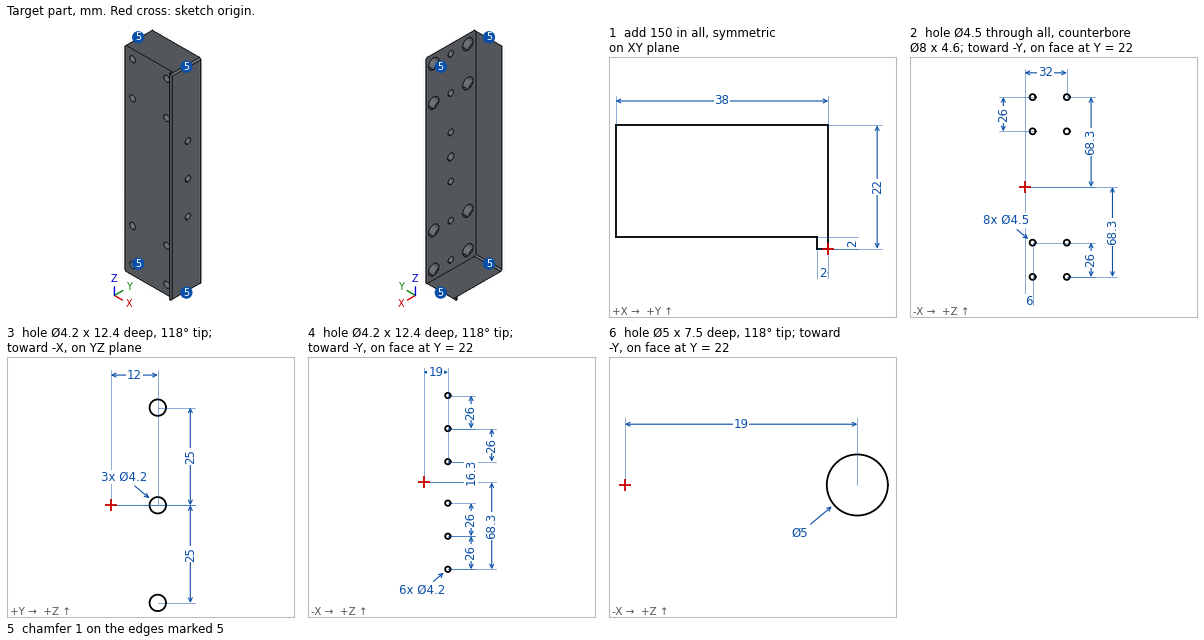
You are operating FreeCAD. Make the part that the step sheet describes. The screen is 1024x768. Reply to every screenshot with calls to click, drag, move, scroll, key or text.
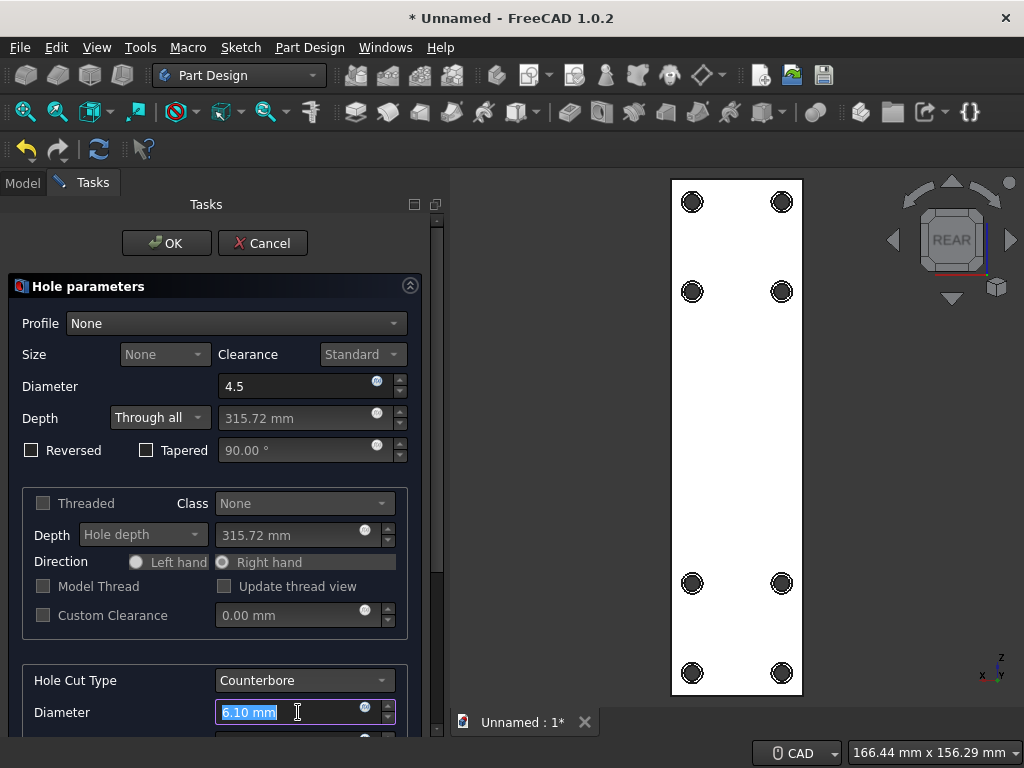
text(8)
key(Tab)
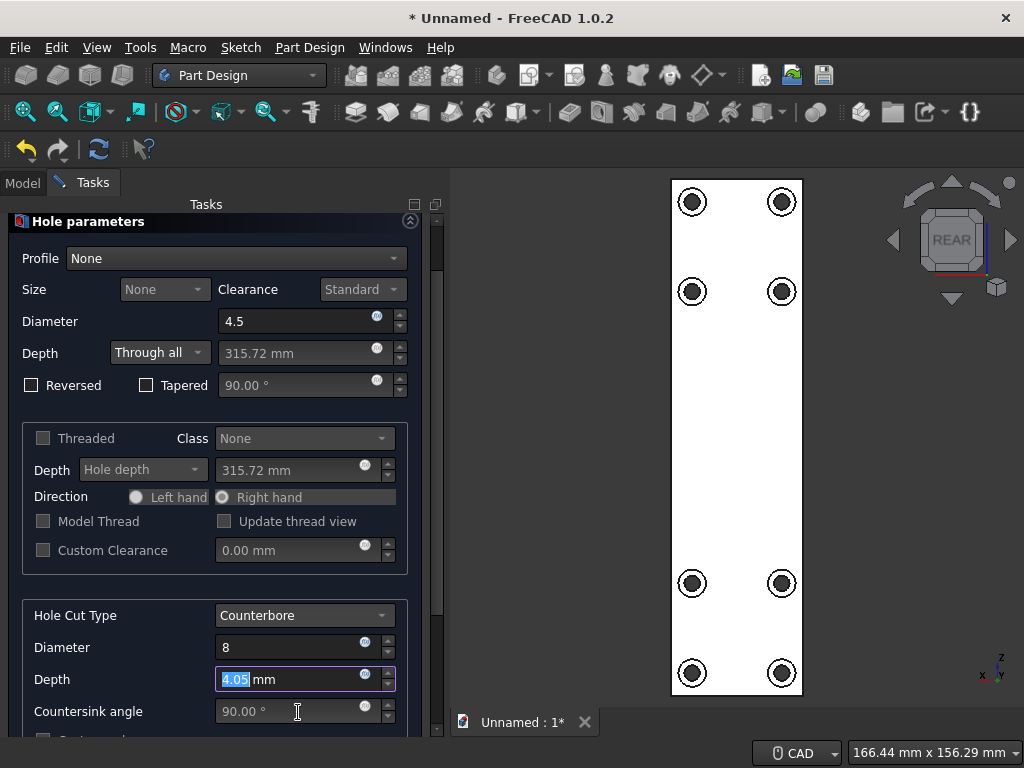
text(4.6)
key(Tab)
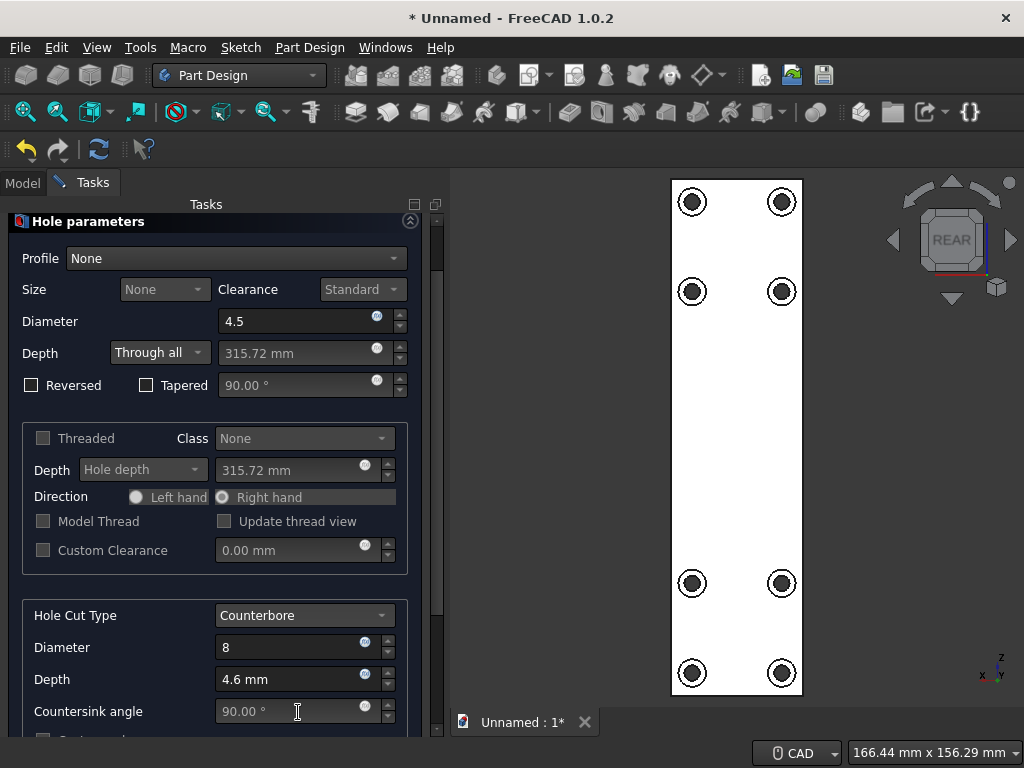
scroll(437, 475, up, 2)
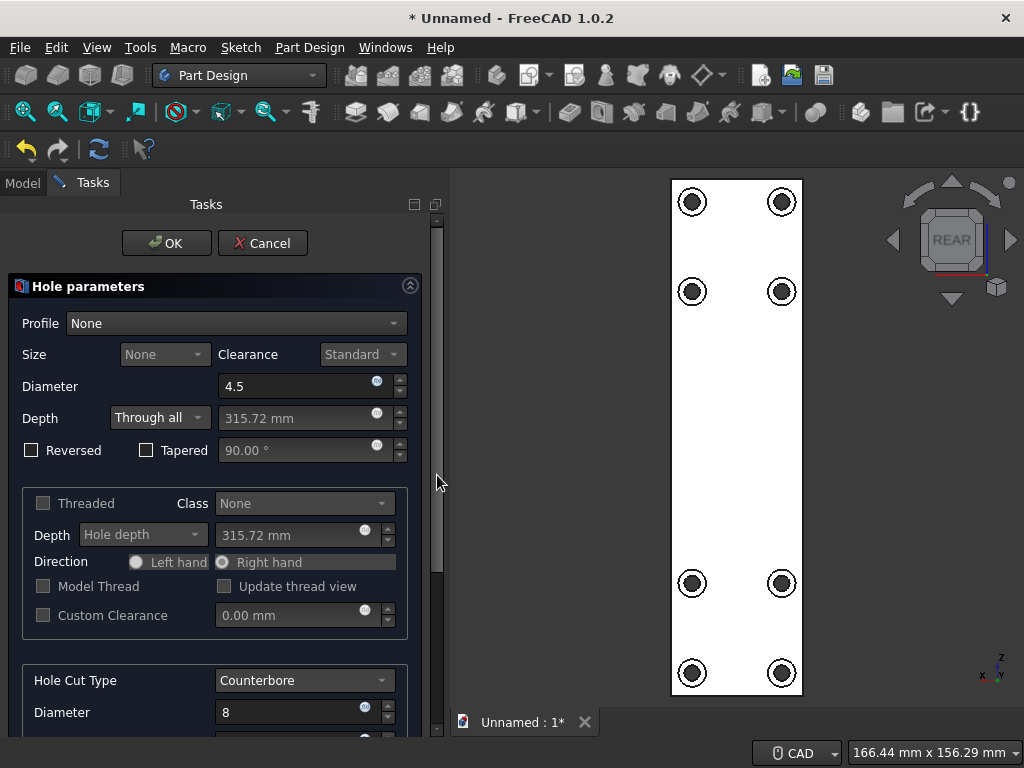
click(167, 243)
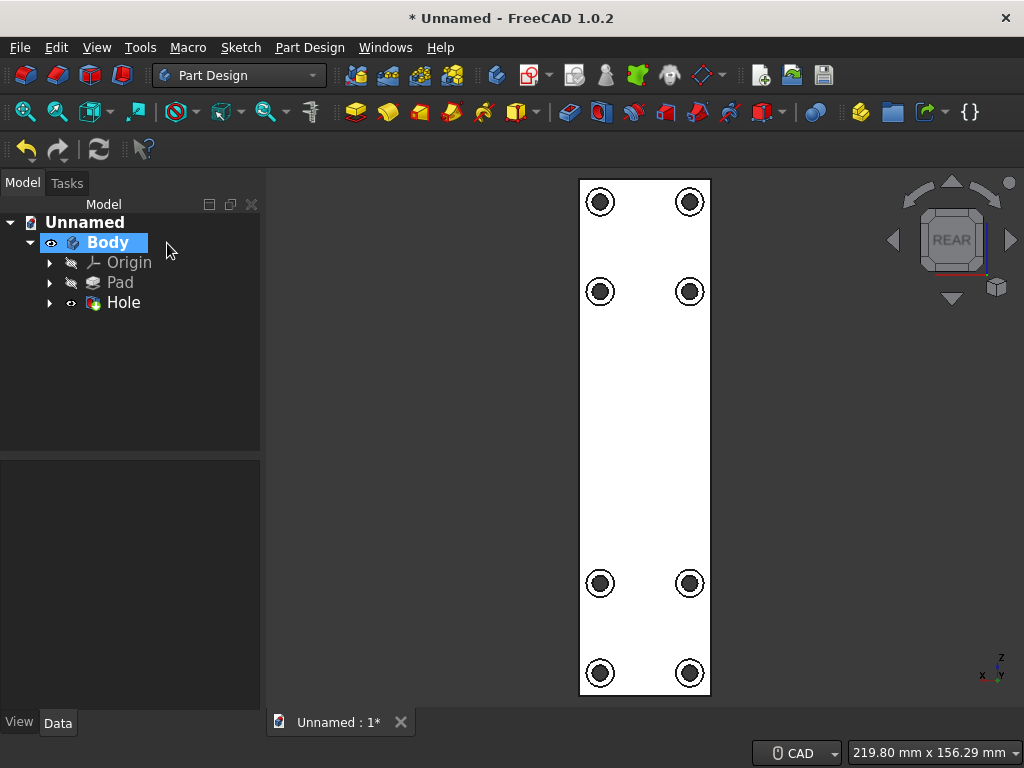
click(530, 76)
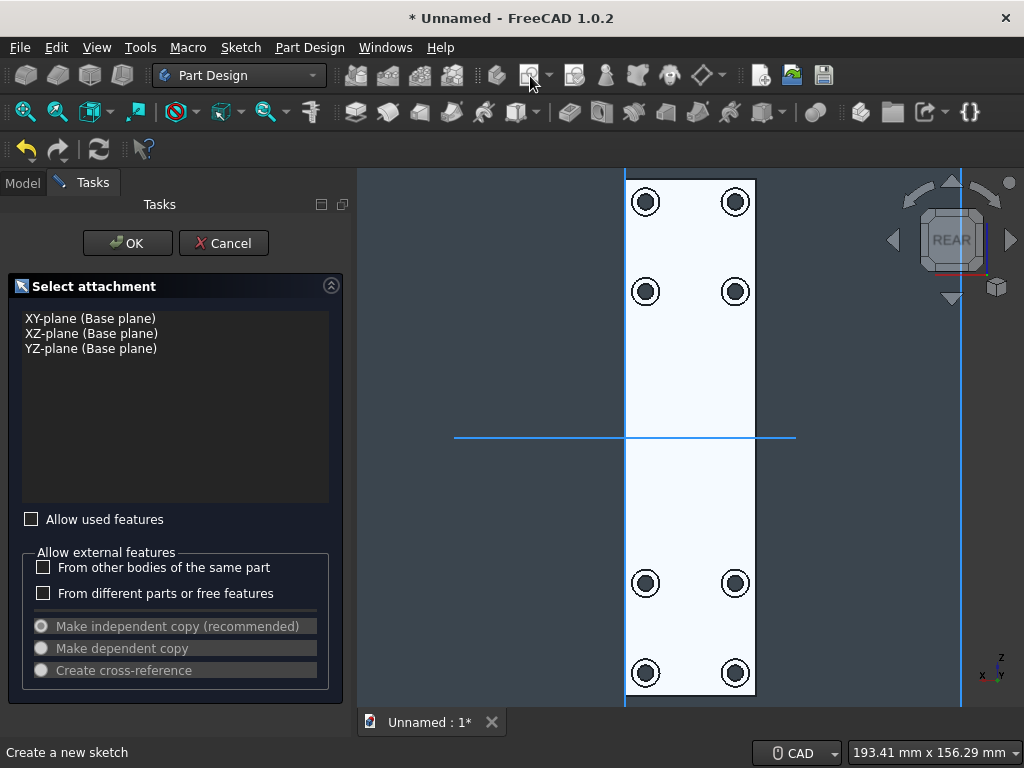
click(82, 348)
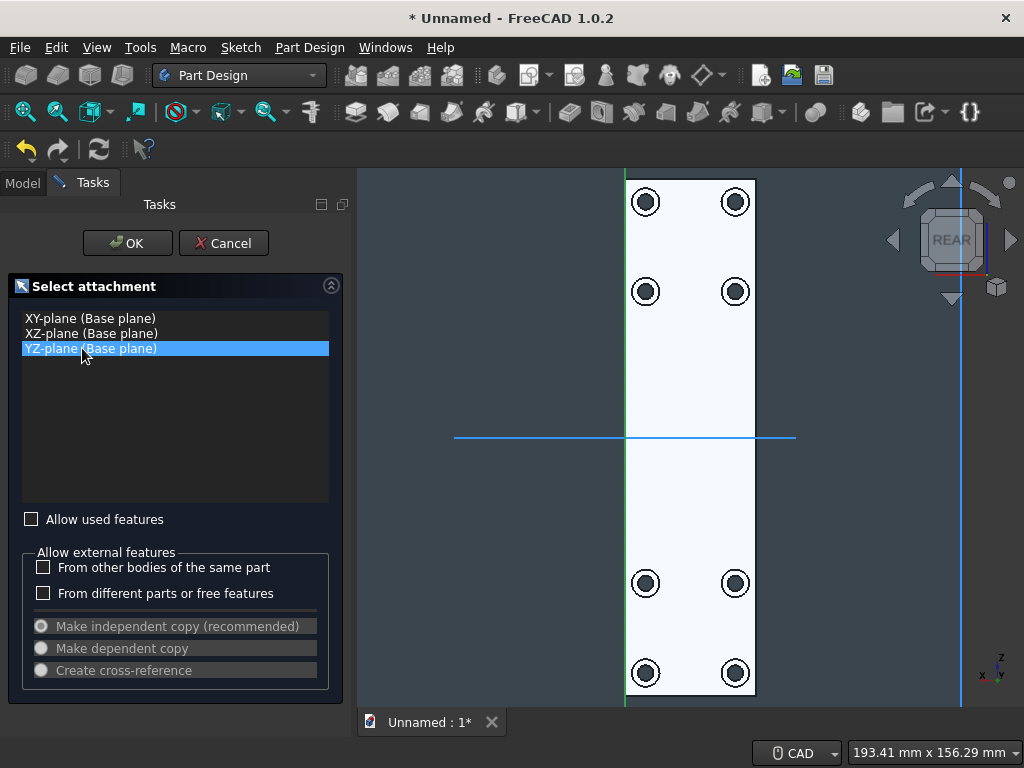
click(128, 243)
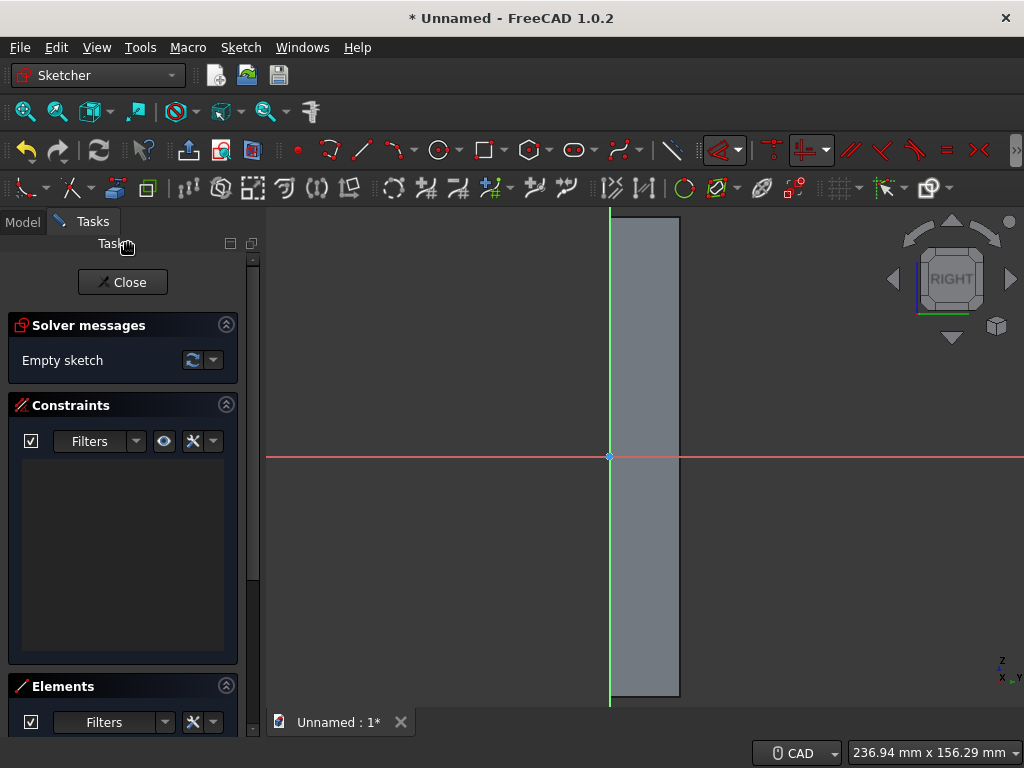
scroll(700, 457, up, 3)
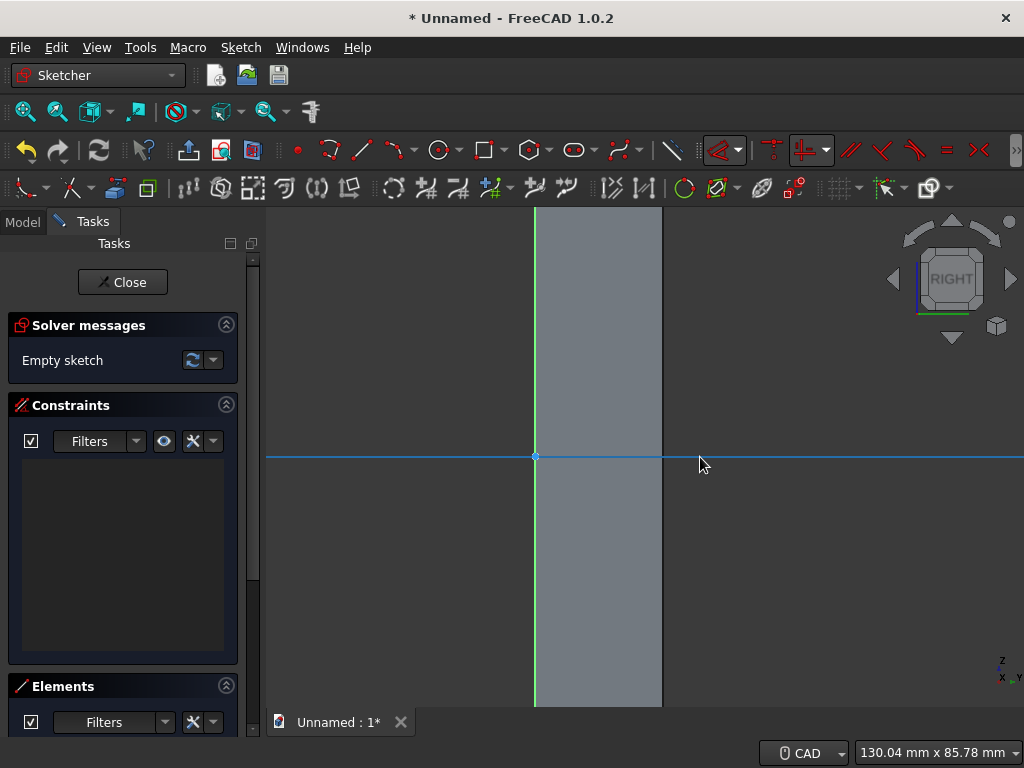
click(440, 150)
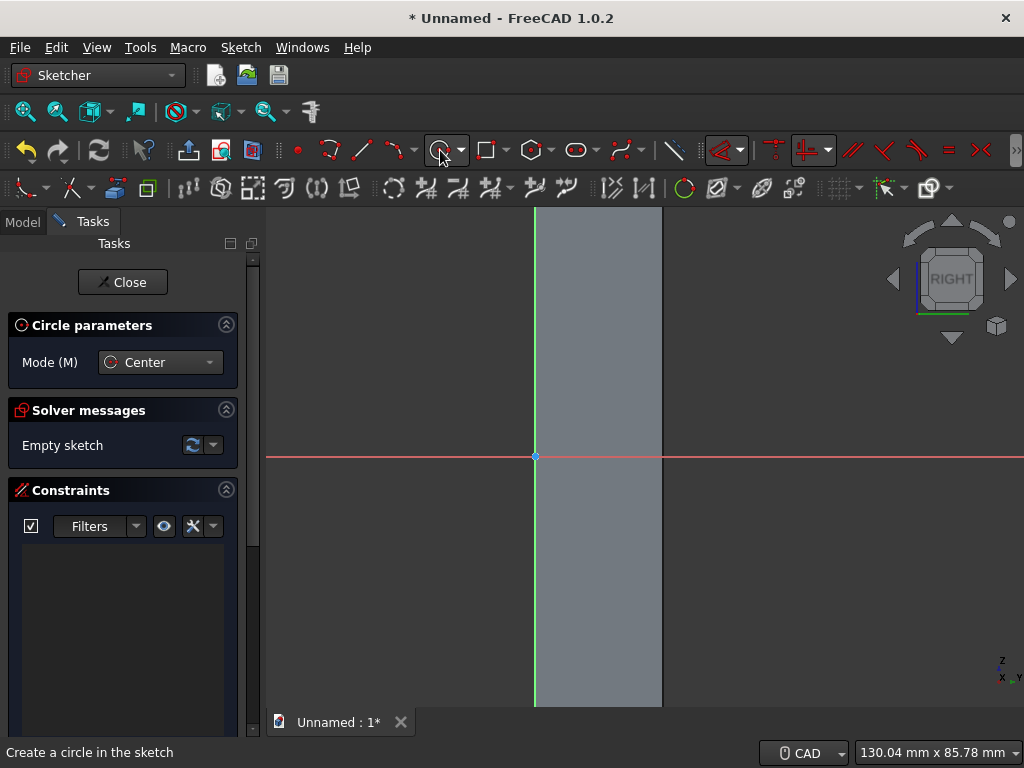
scroll(605, 457, up, 4)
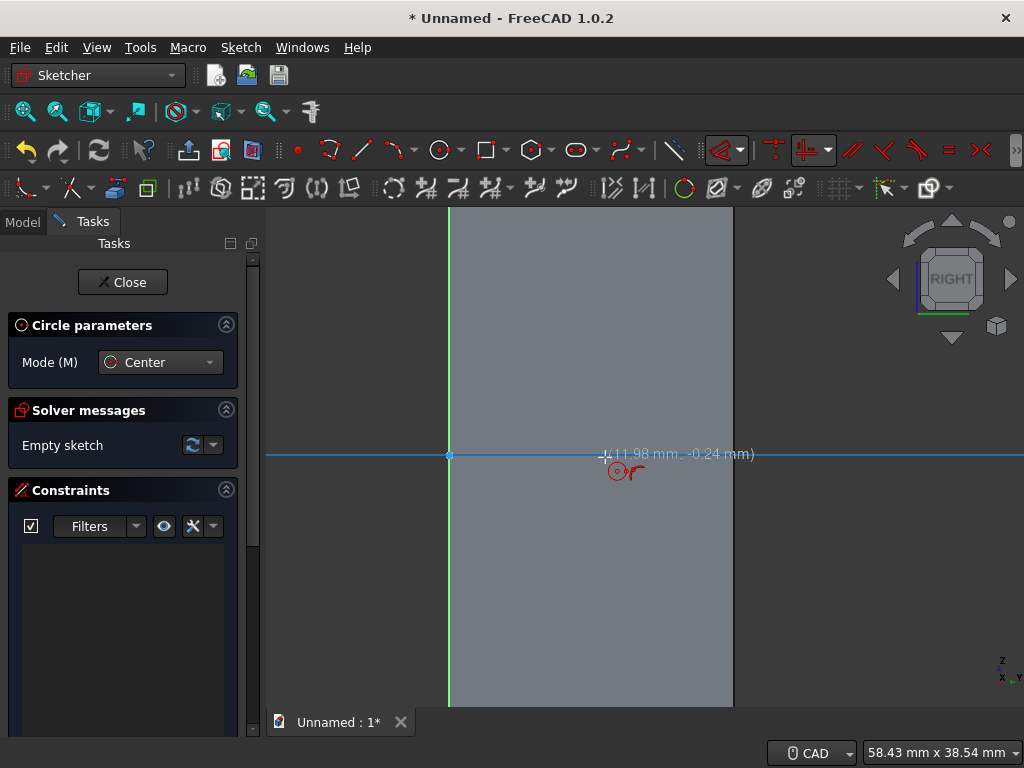
click(605, 455)
click(624, 436)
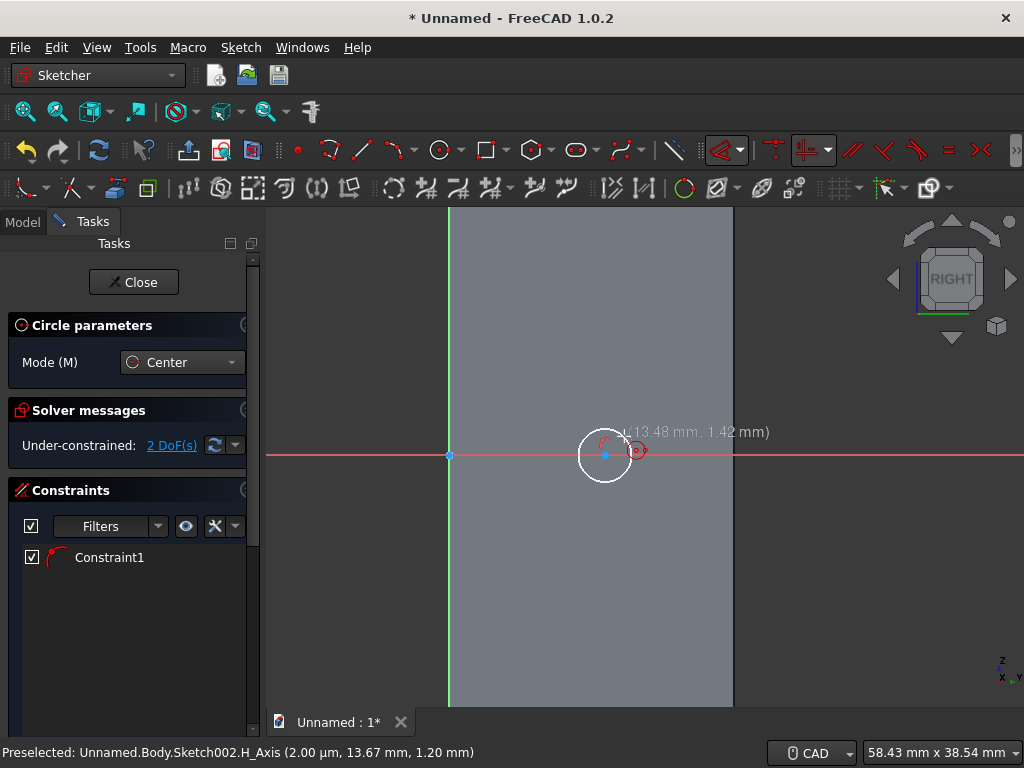
scroll(606, 458, down, 4)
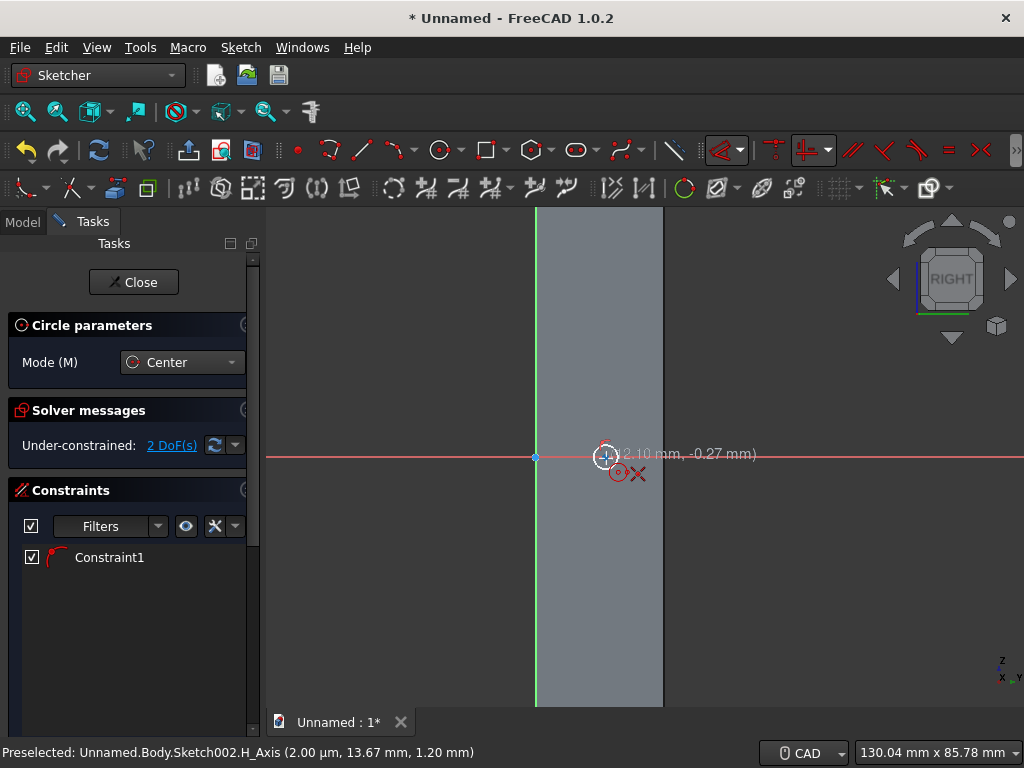
scroll(606, 311, up, 4)